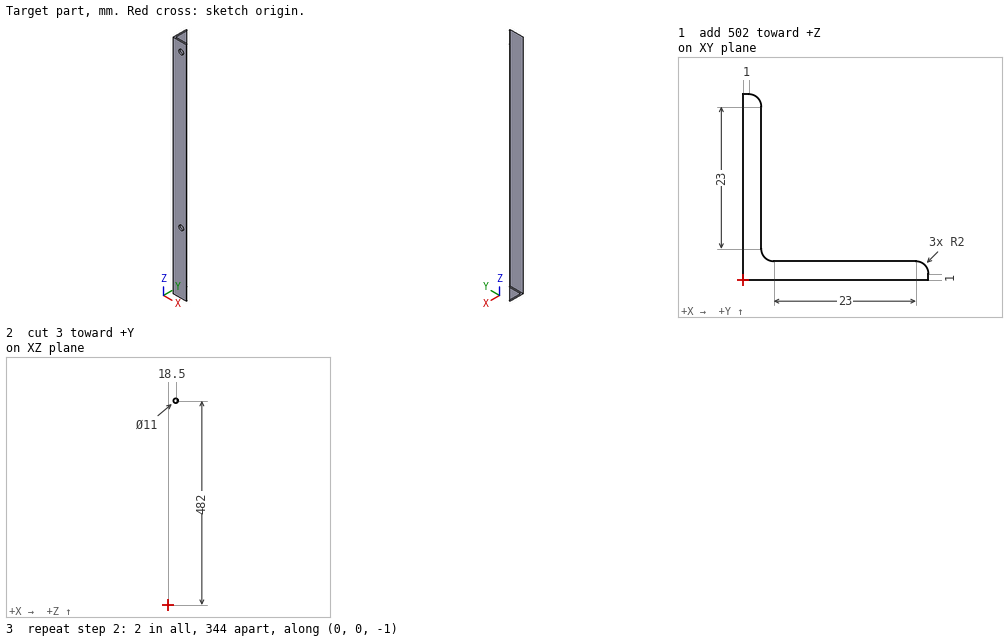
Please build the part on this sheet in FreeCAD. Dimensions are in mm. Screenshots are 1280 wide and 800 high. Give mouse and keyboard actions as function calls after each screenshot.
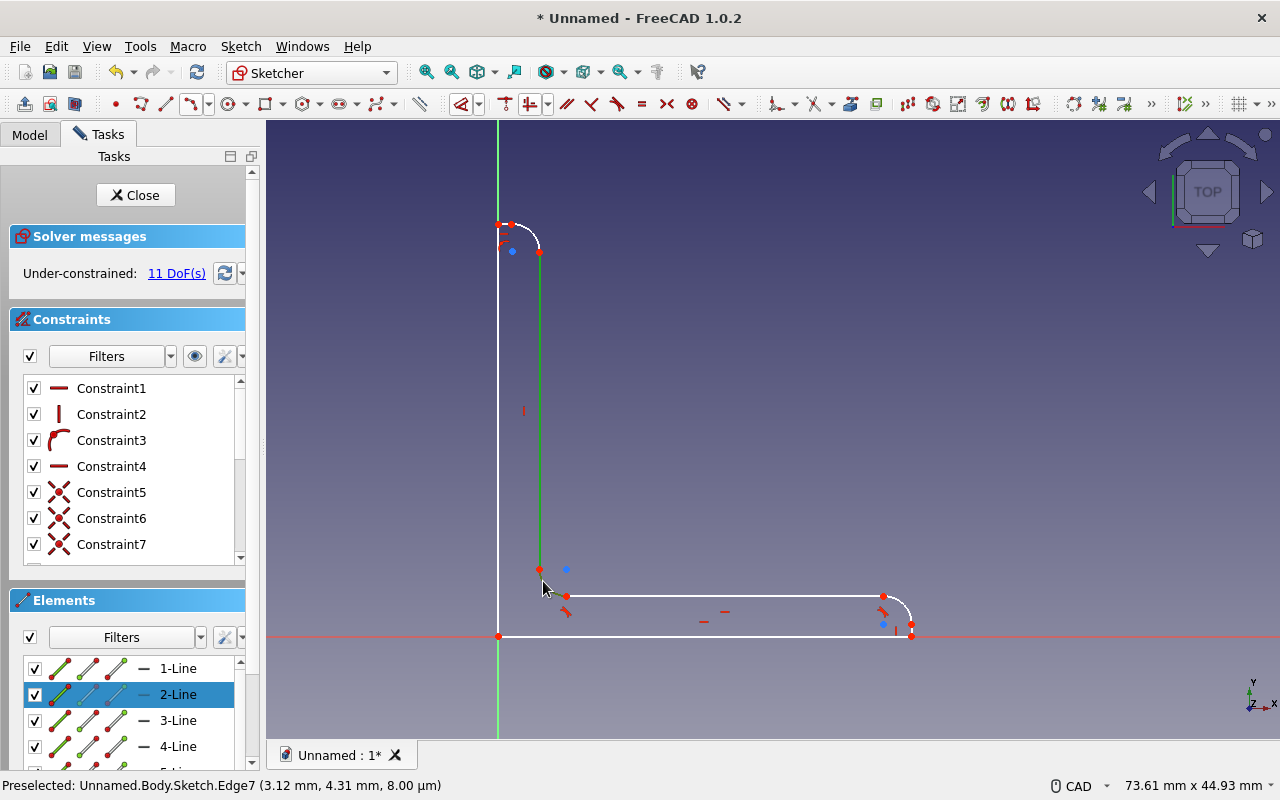
click(617, 104)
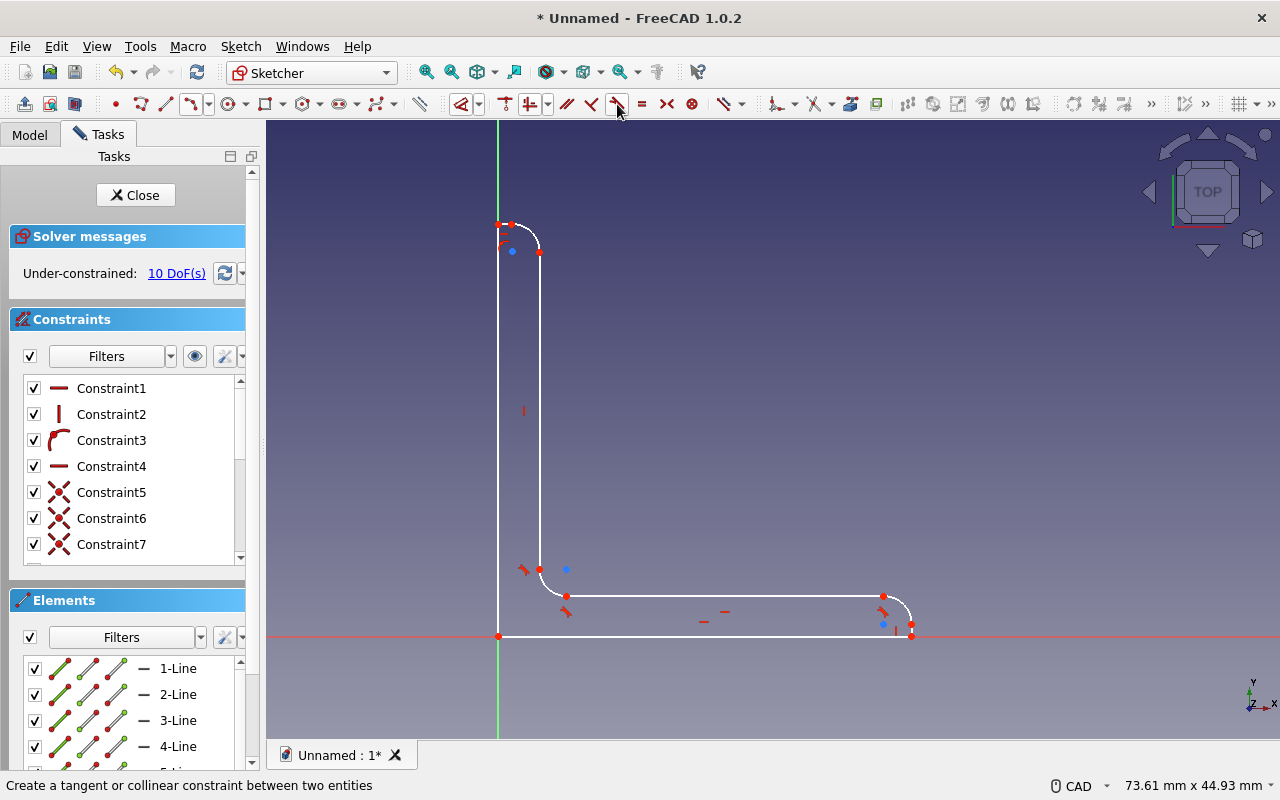
click(540, 474)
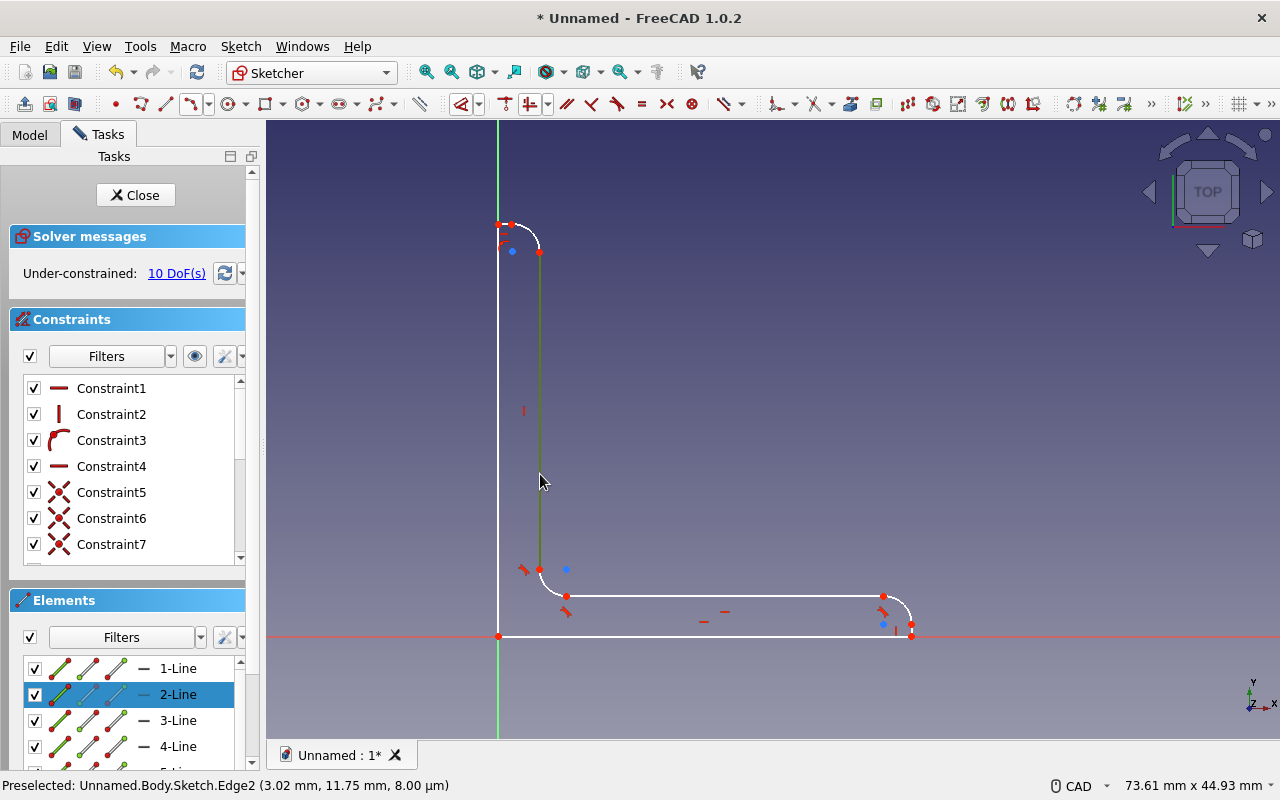
click(537, 239)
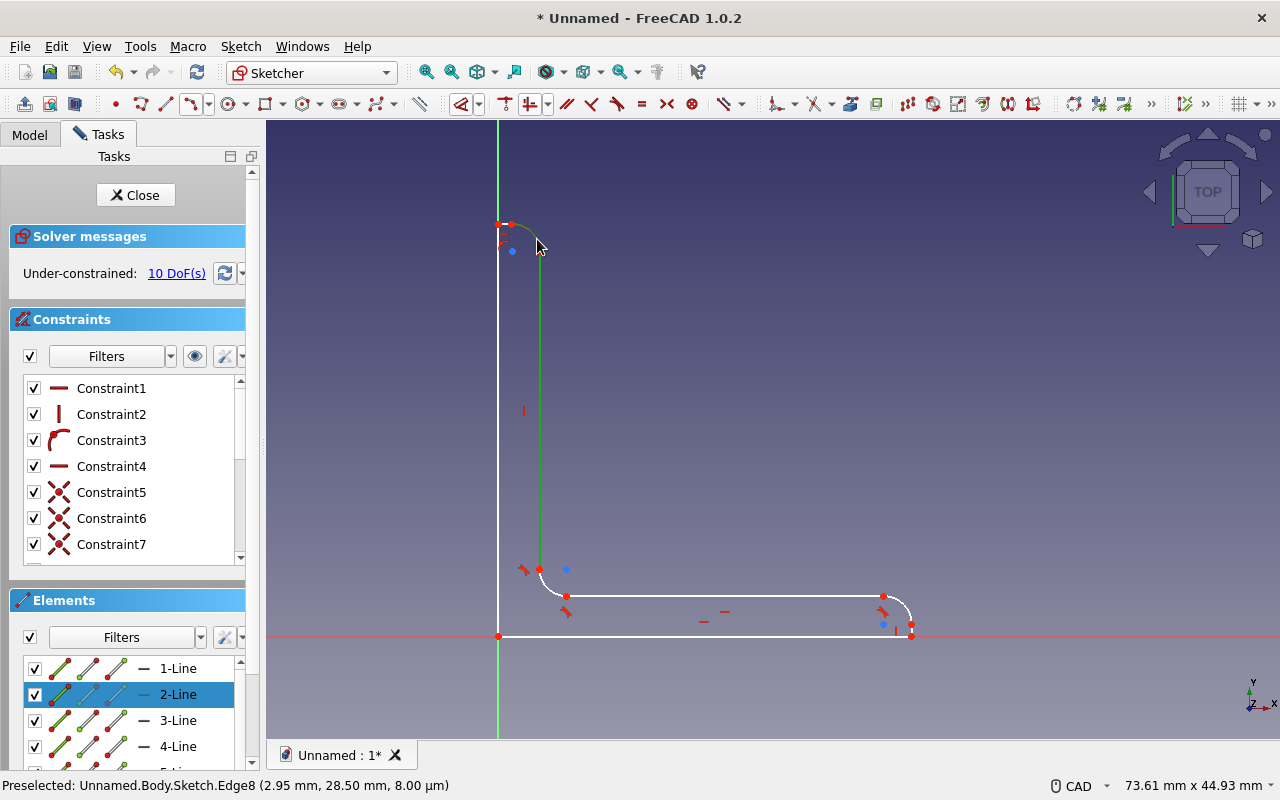
click(617, 104)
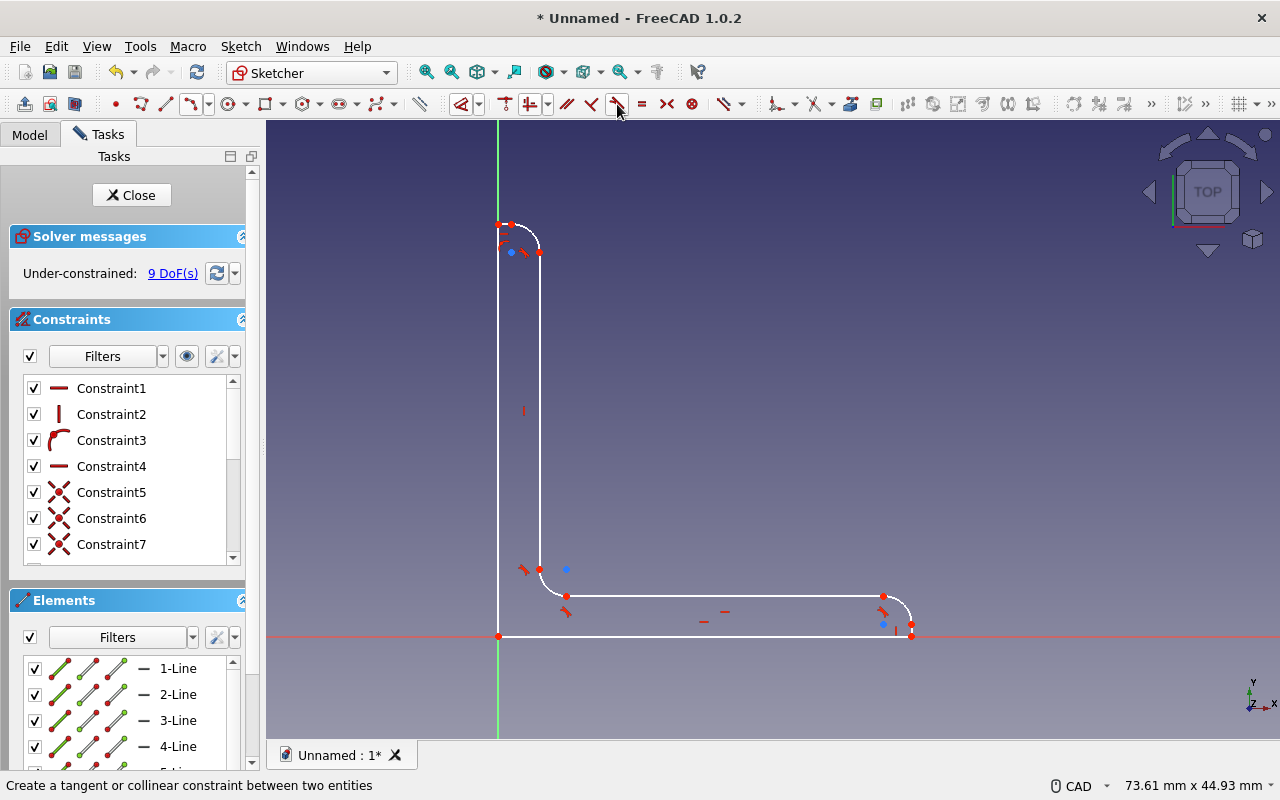
scroll(505, 224, up, 4)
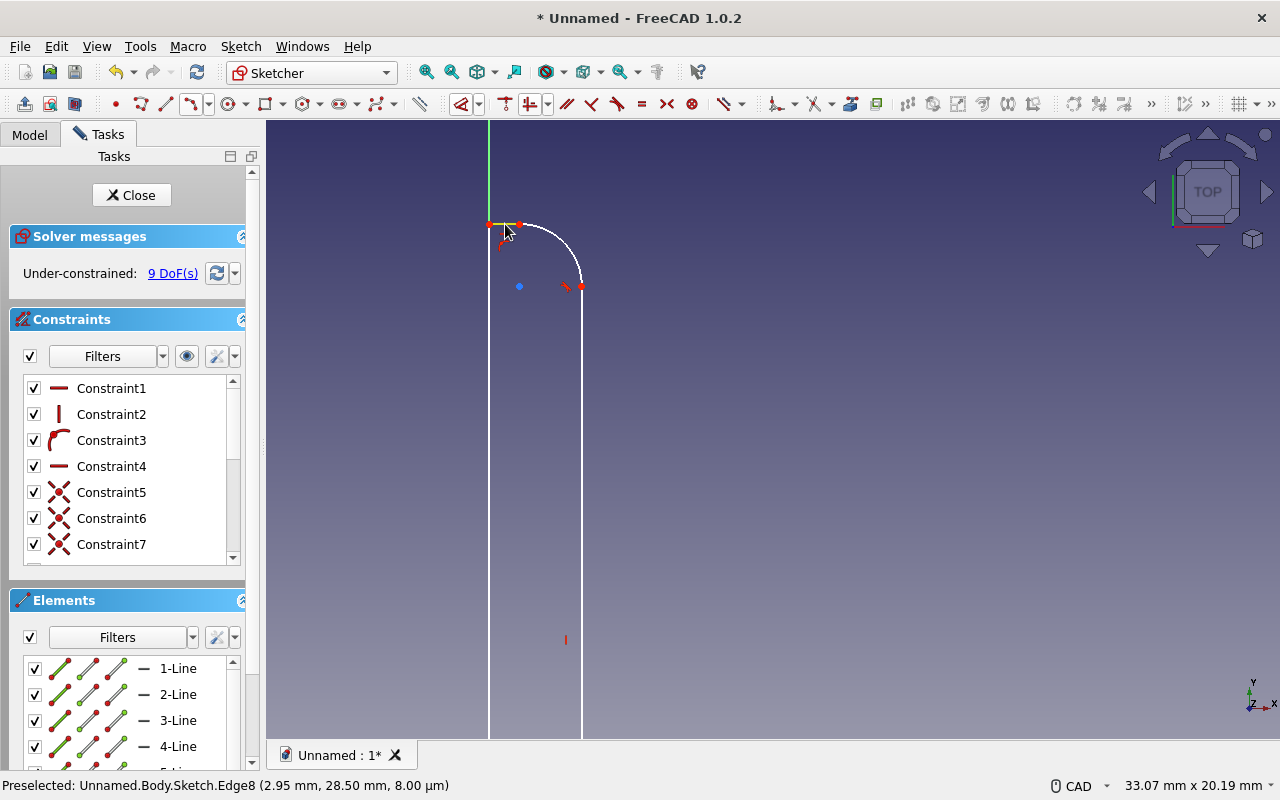
click(504, 224)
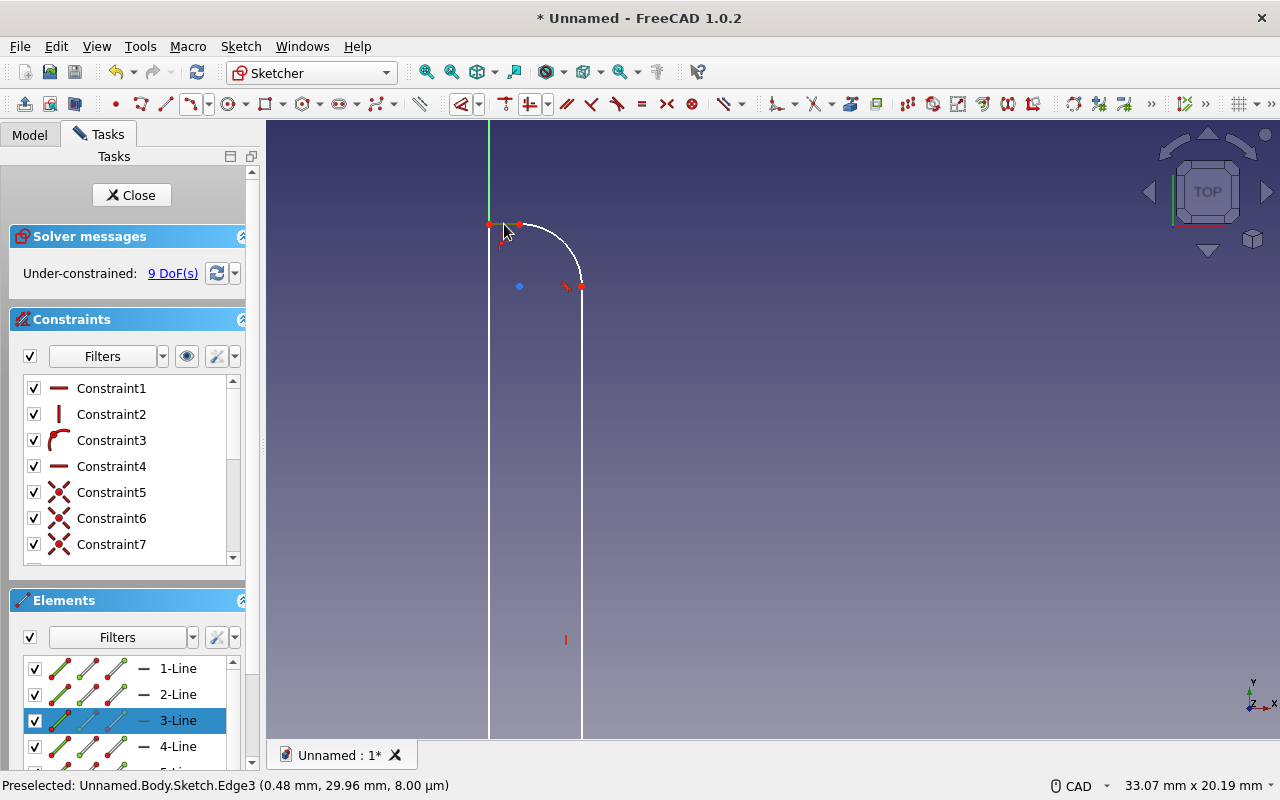
click(575, 258)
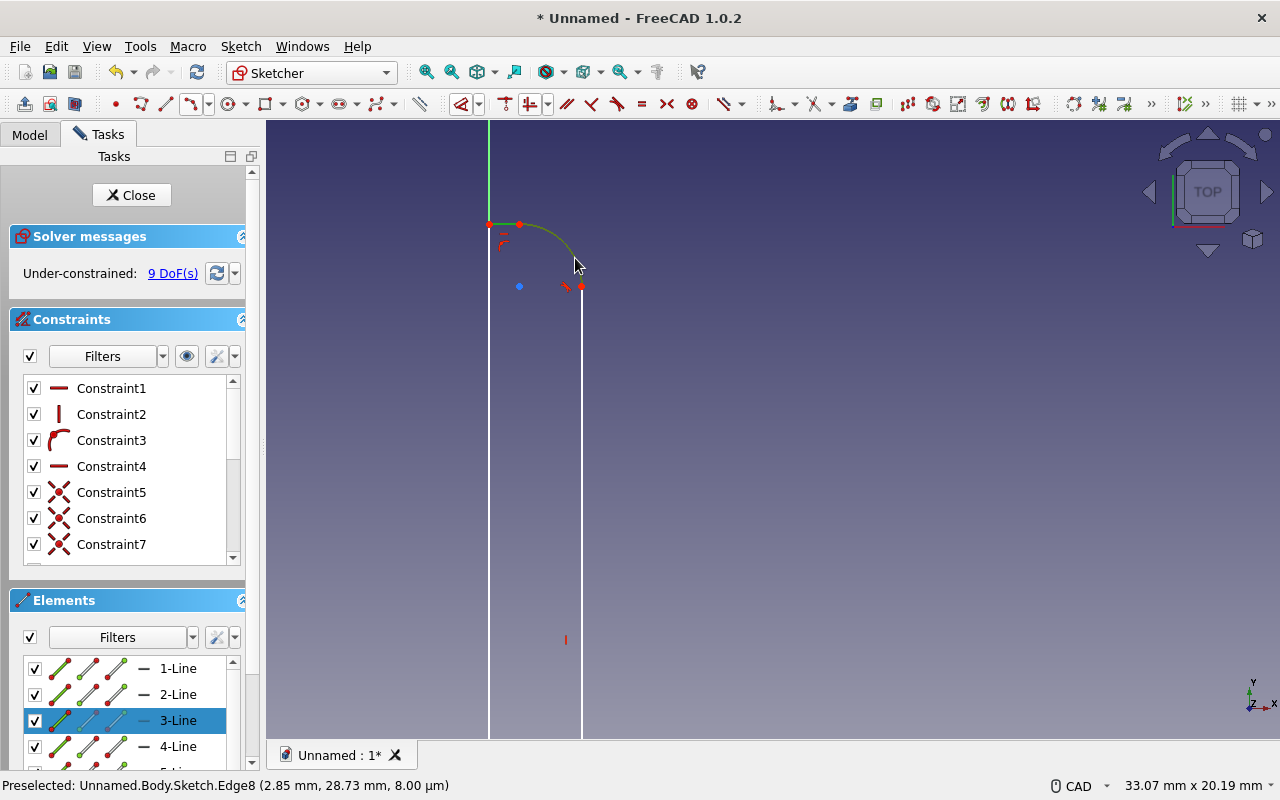
key(t)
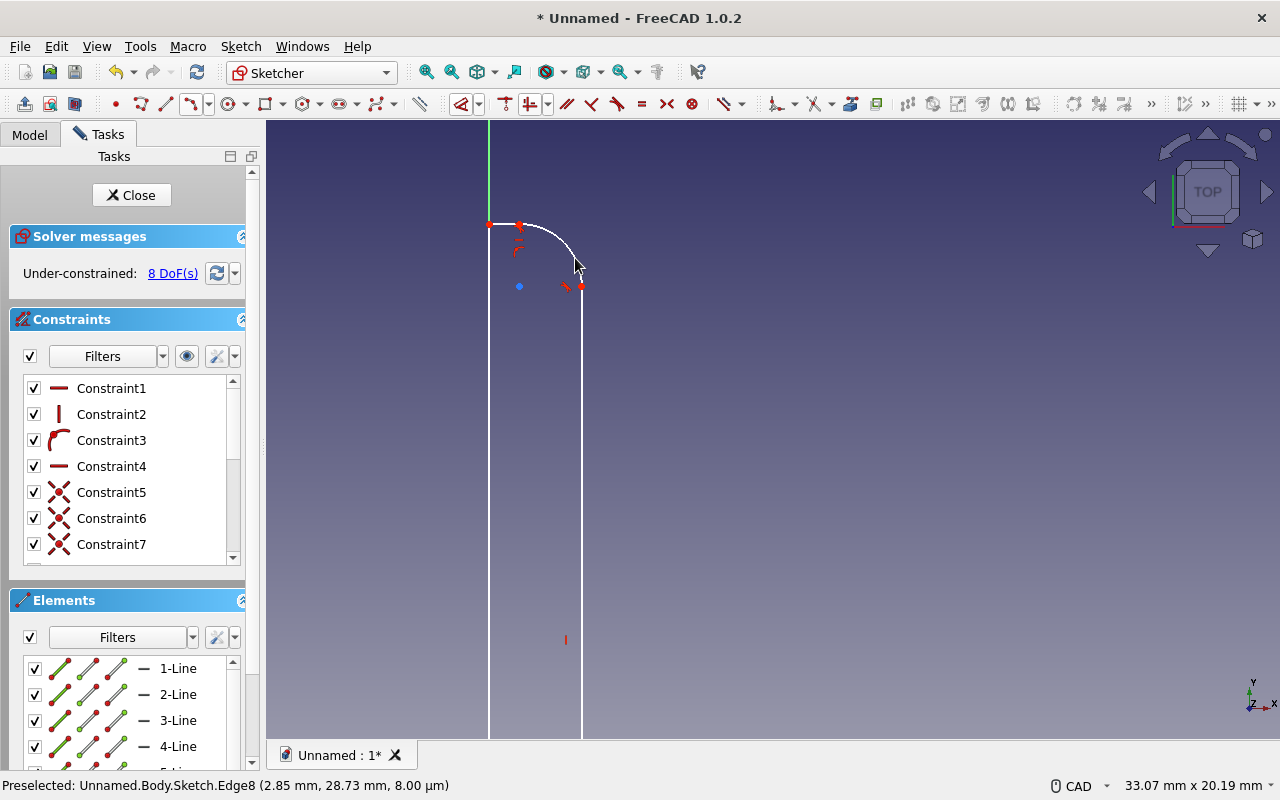
scroll(505, 223, down, 4)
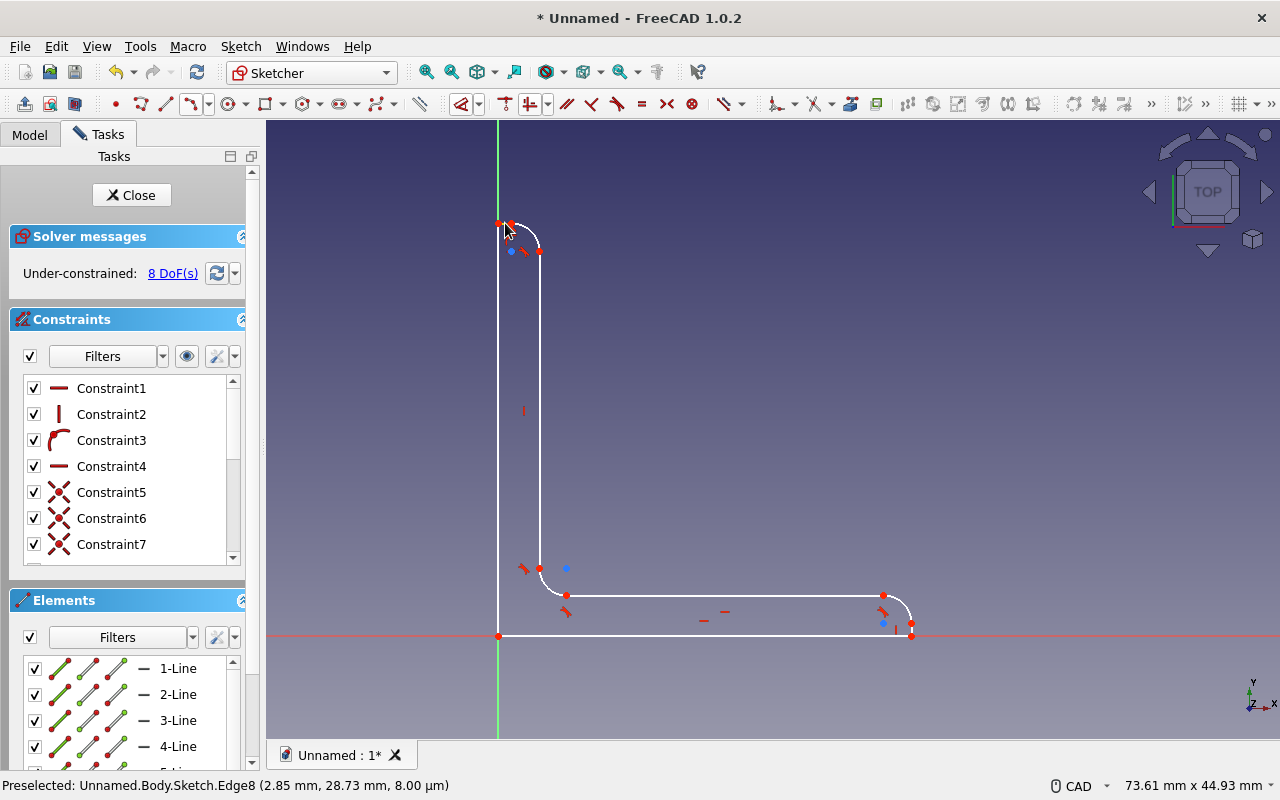
scroll(912, 631, up, 5)